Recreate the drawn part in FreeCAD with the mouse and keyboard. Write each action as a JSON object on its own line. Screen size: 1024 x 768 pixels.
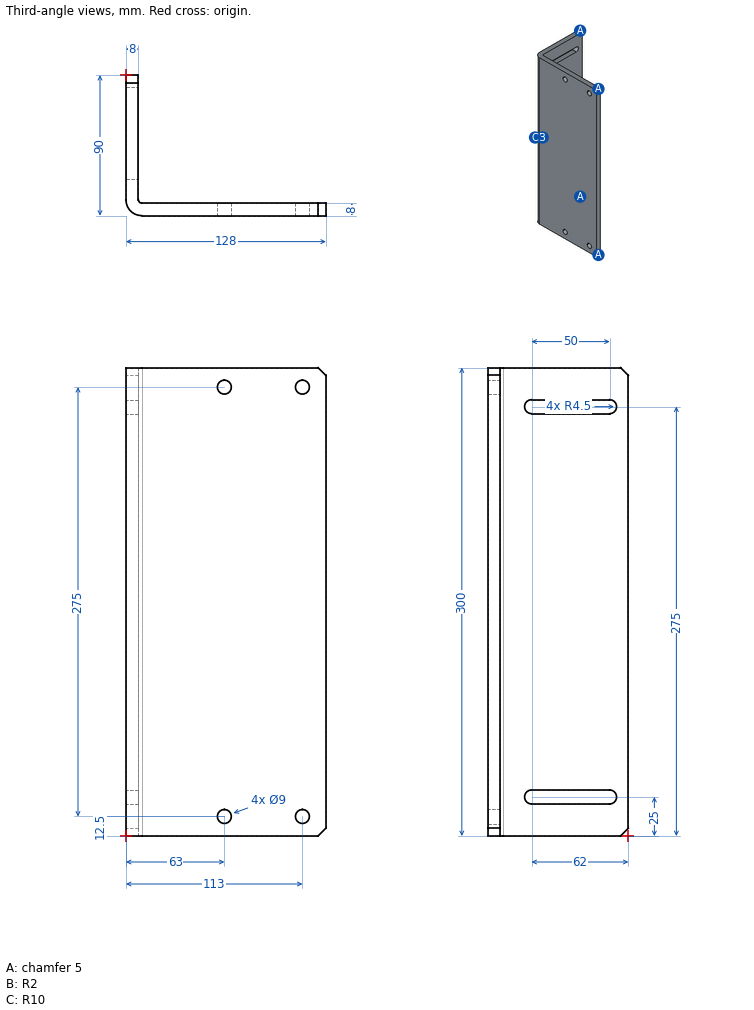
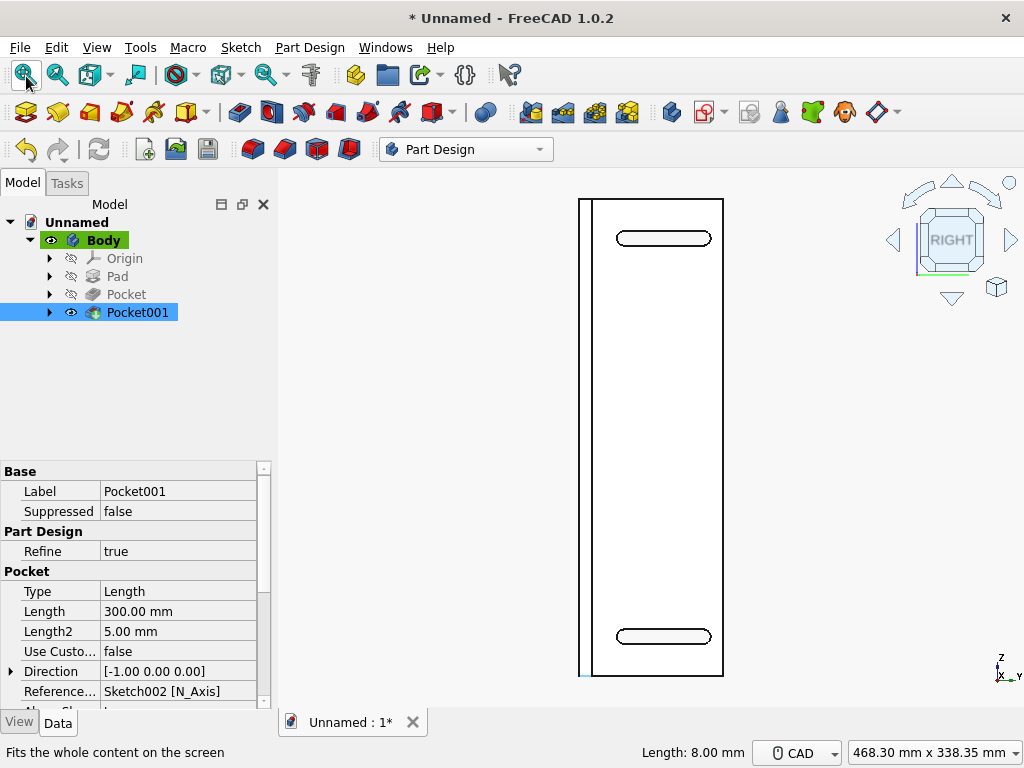
{"action": "key", "text": "0"}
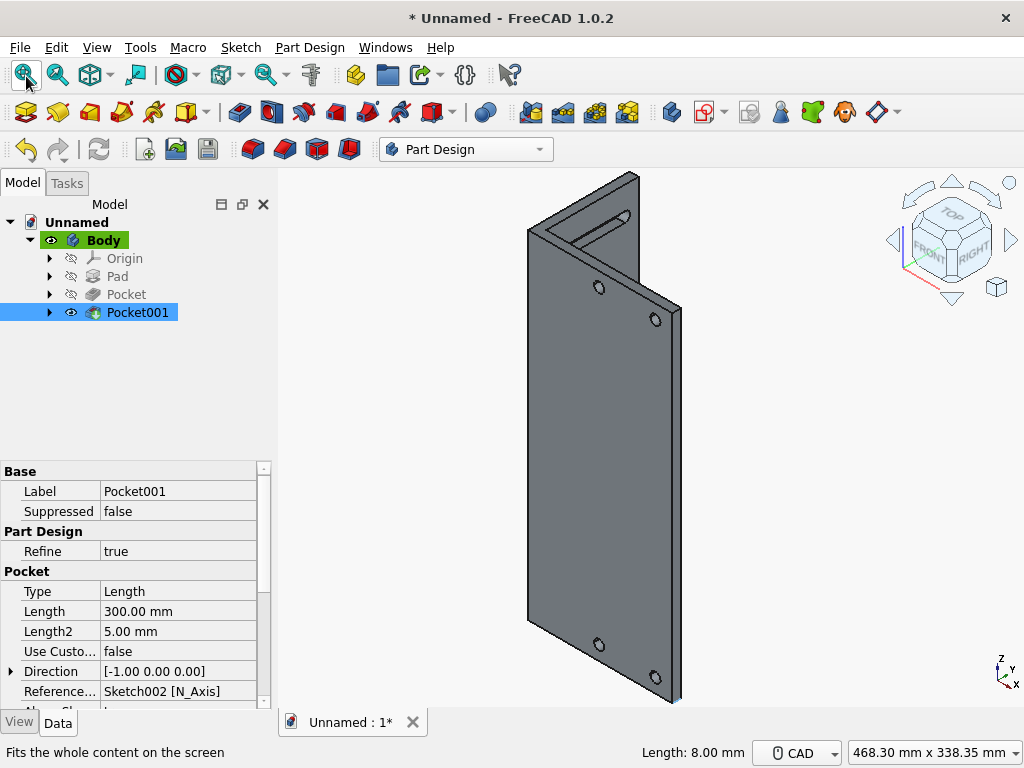
{"action": "left_click", "coordinate": [678, 309], "text": "ctrl"}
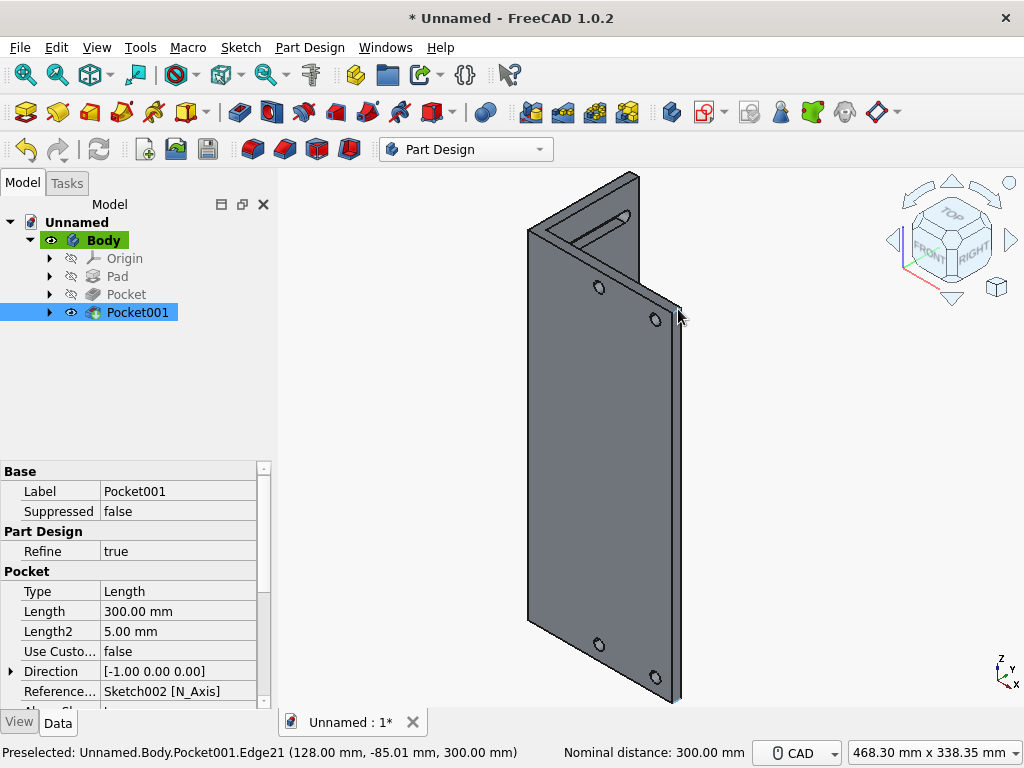
{"action": "key", "text": "2"}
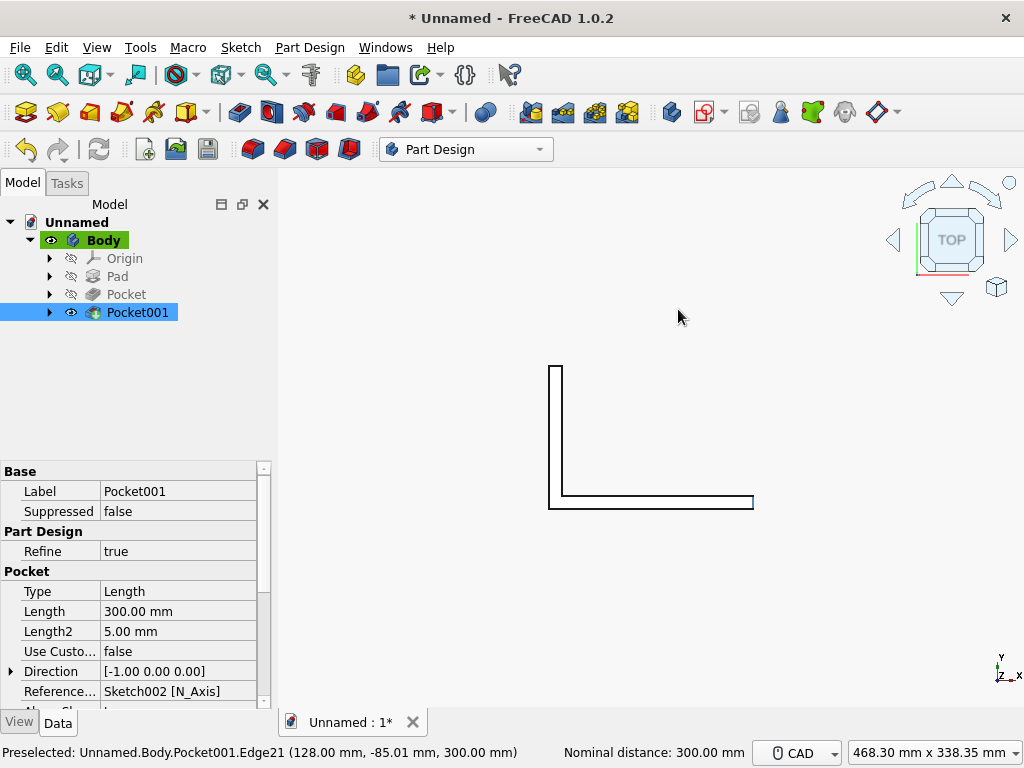
{"action": "left_click", "coordinate": [26, 76]}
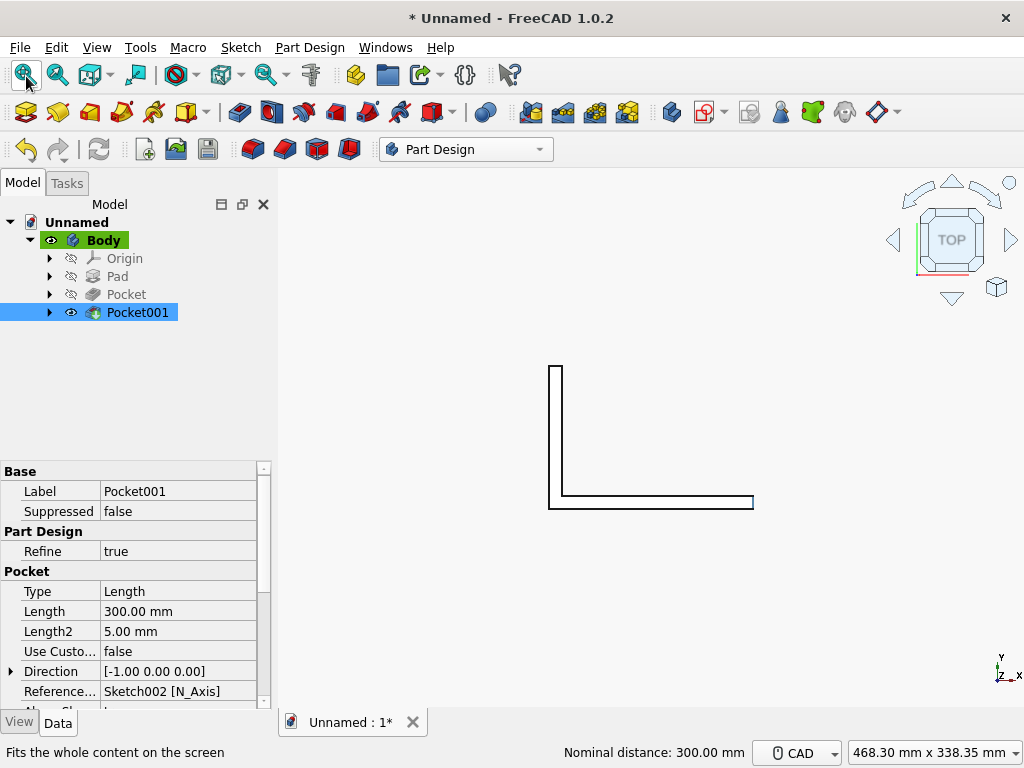
{"action": "scroll", "coordinate": [555, 365], "scroll_direction": "up", "scroll_amount": 6}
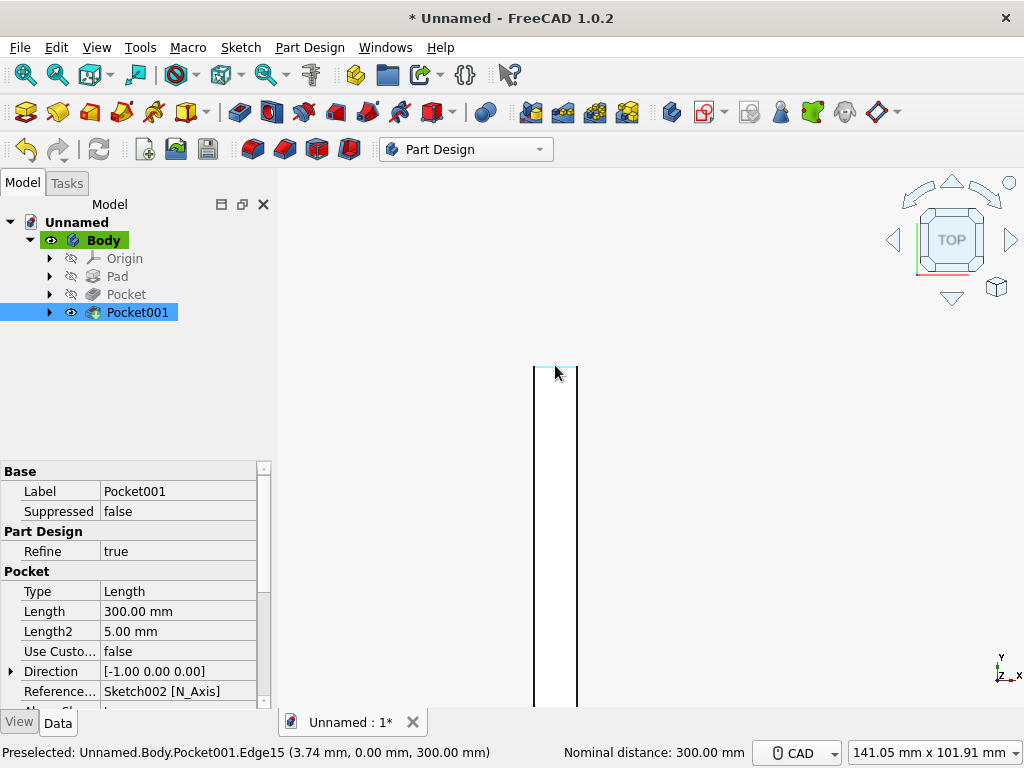
{"action": "left_click", "coordinate": [556, 366], "text": "ctrl"}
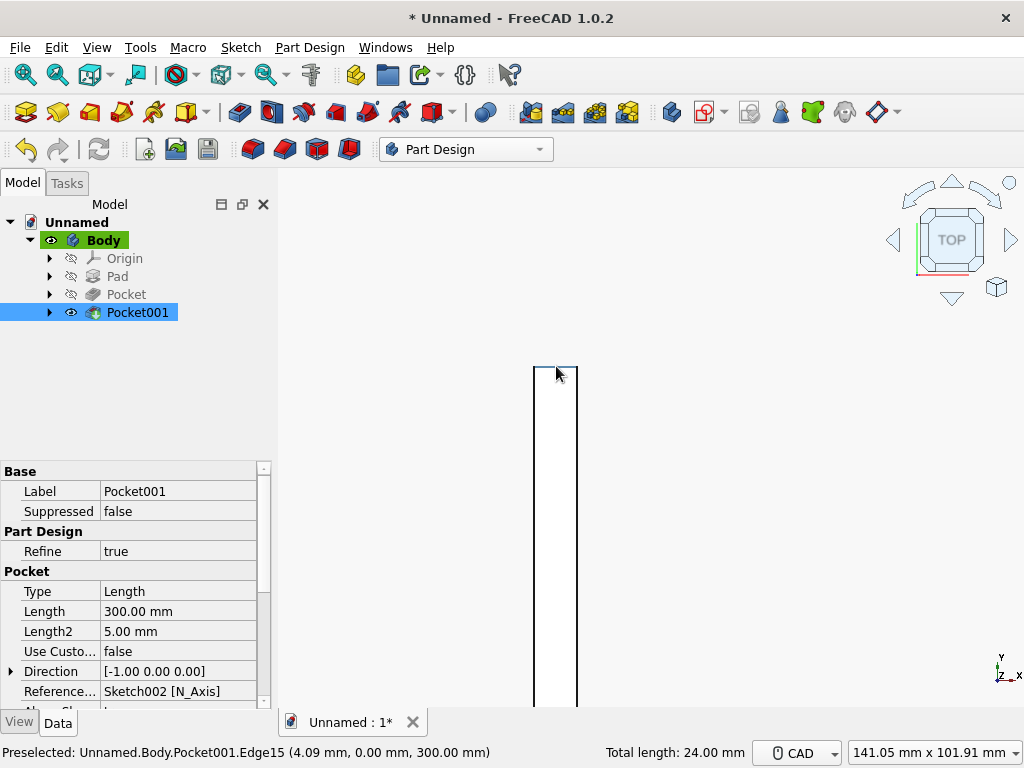
{"action": "left_click", "coordinate": [26, 76]}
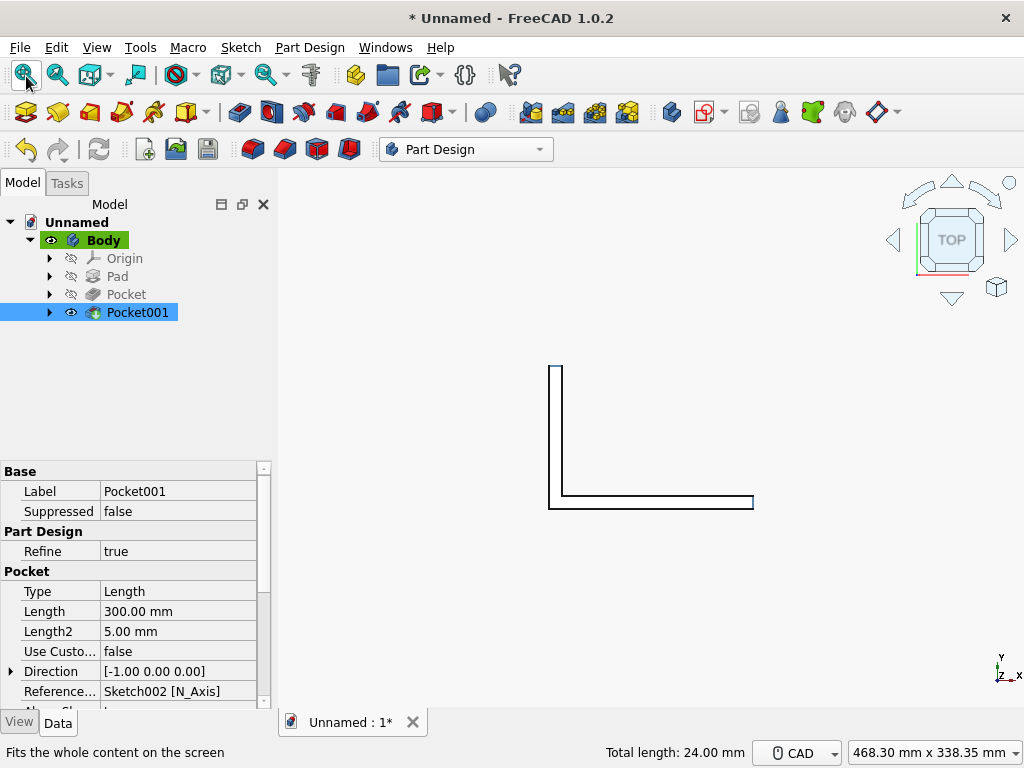
{"action": "key", "text": "1"}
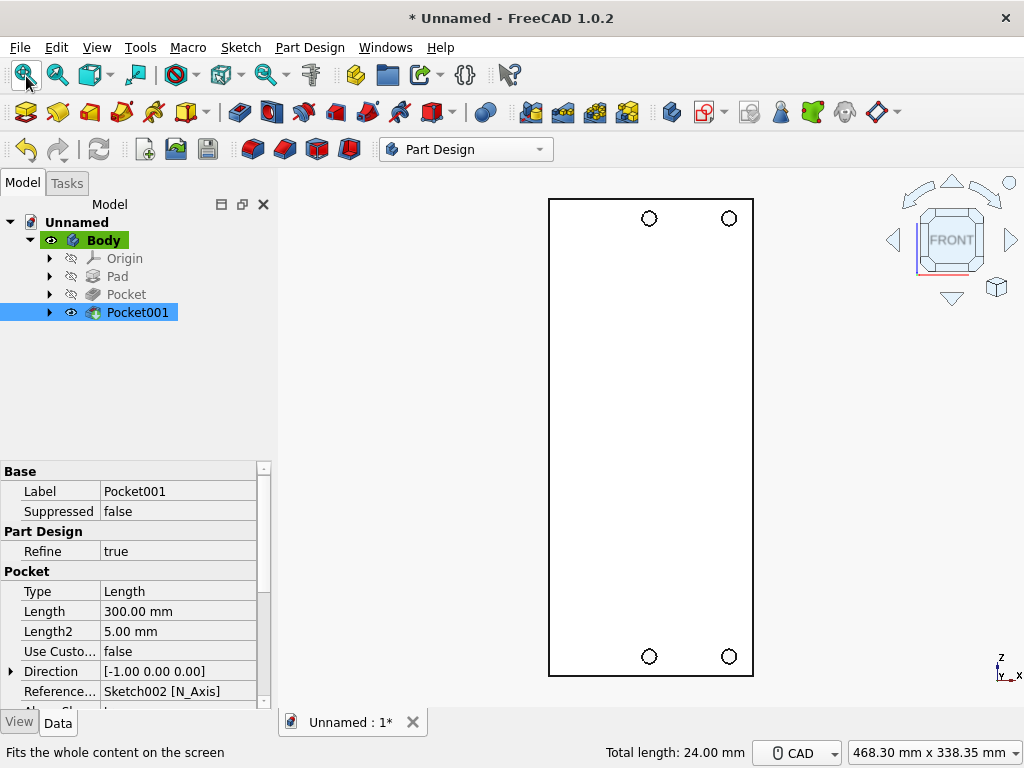
{"action": "scroll", "coordinate": [555, 675], "scroll_direction": "up", "scroll_amount": 6}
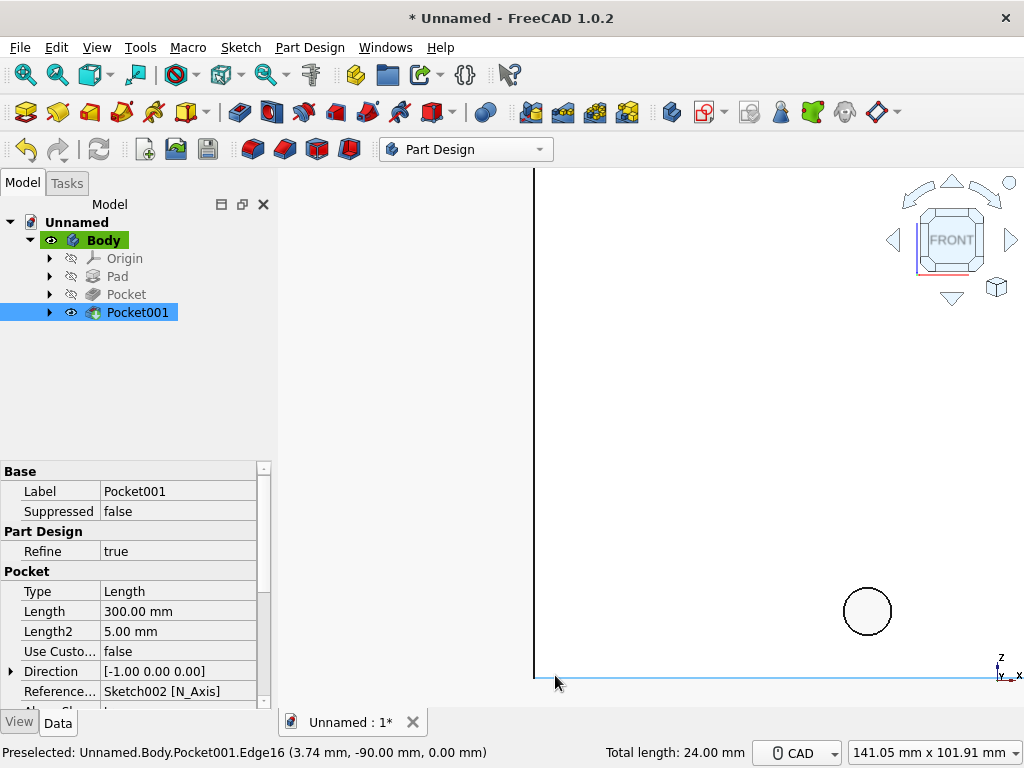
{"action": "left_click", "coordinate": [26, 76]}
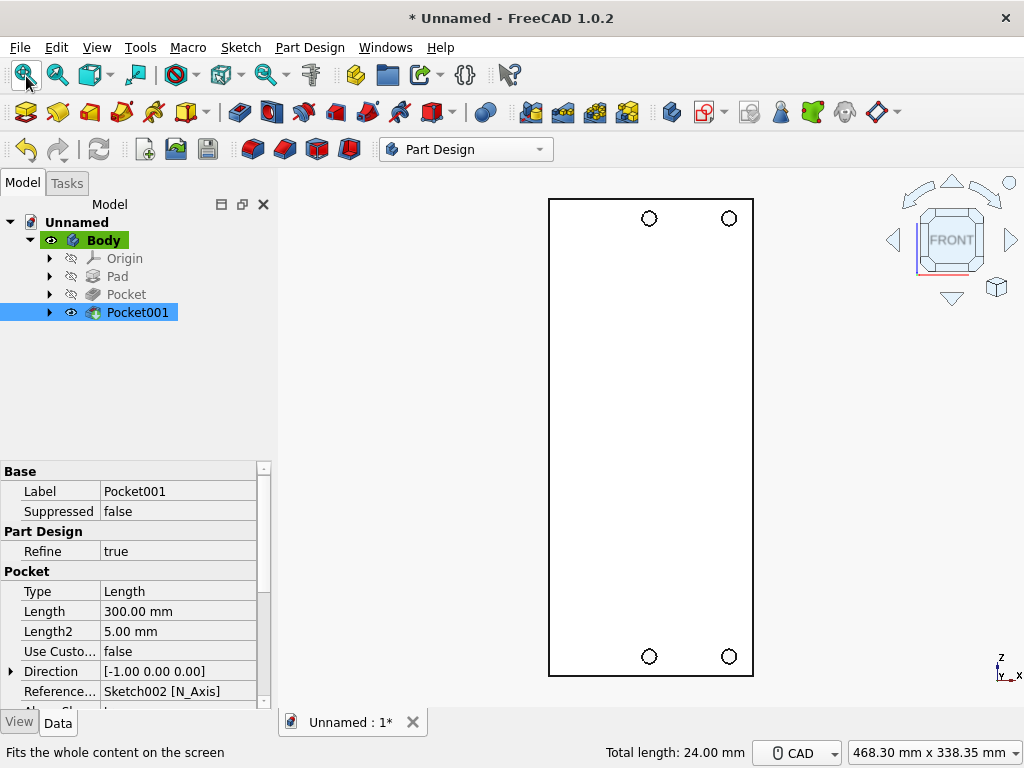
{"action": "key", "text": "3"}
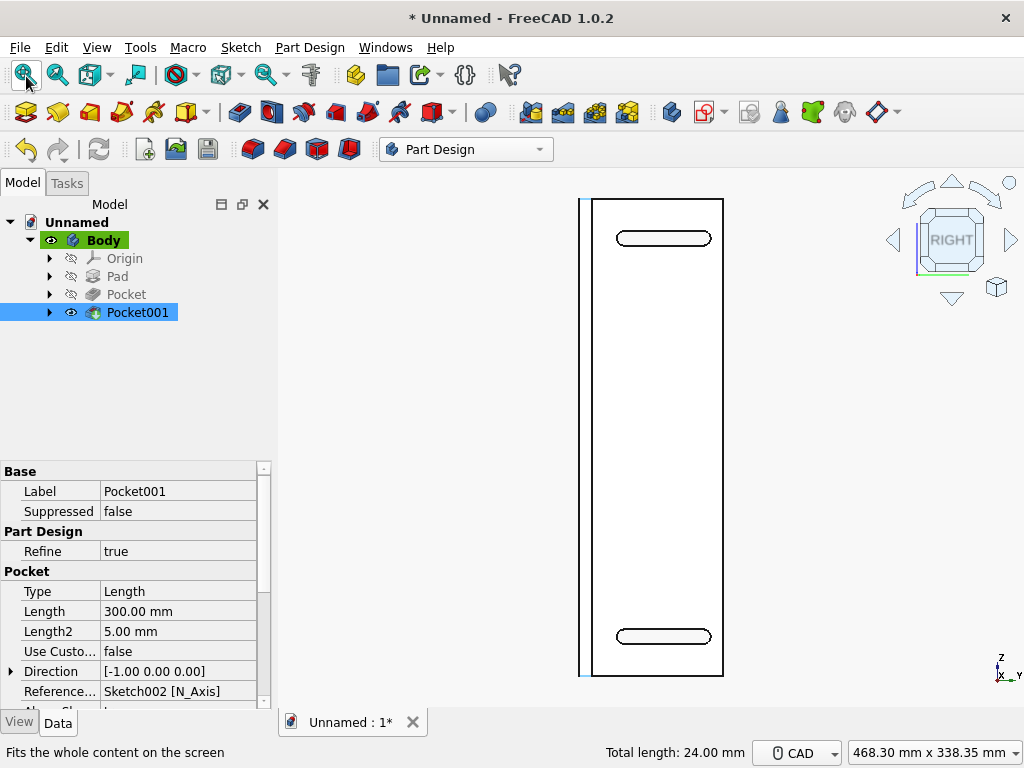
{"action": "scroll", "coordinate": [723, 675], "scroll_direction": "up", "scroll_amount": 6}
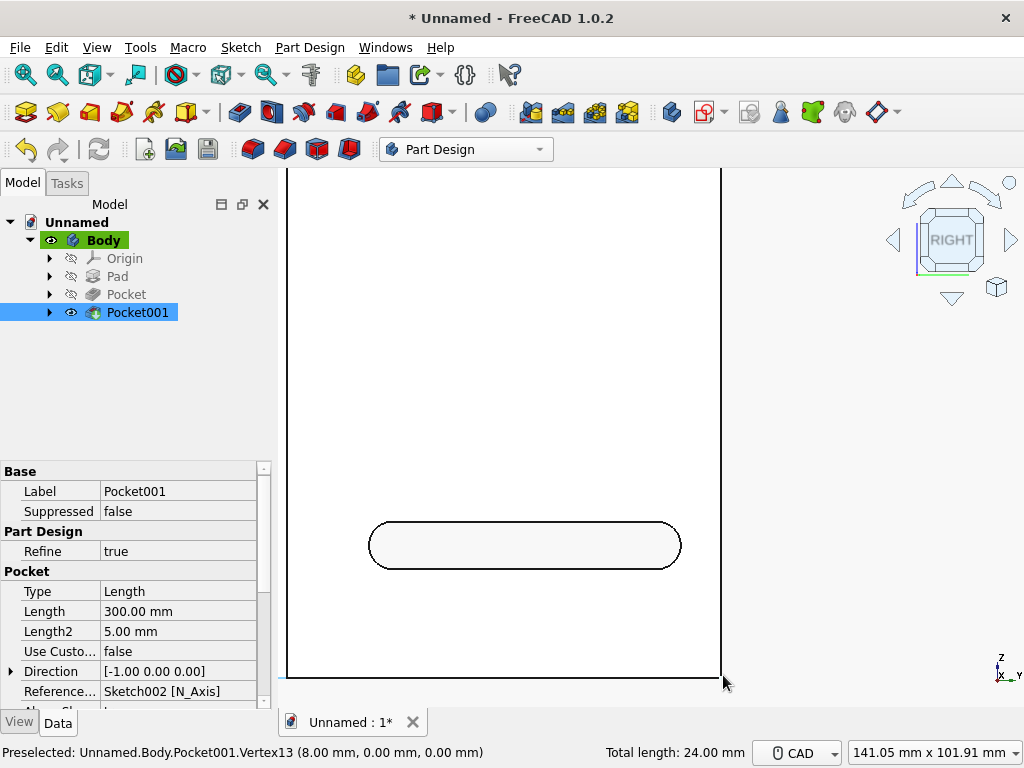
{"action": "left_click", "coordinate": [26, 76]}